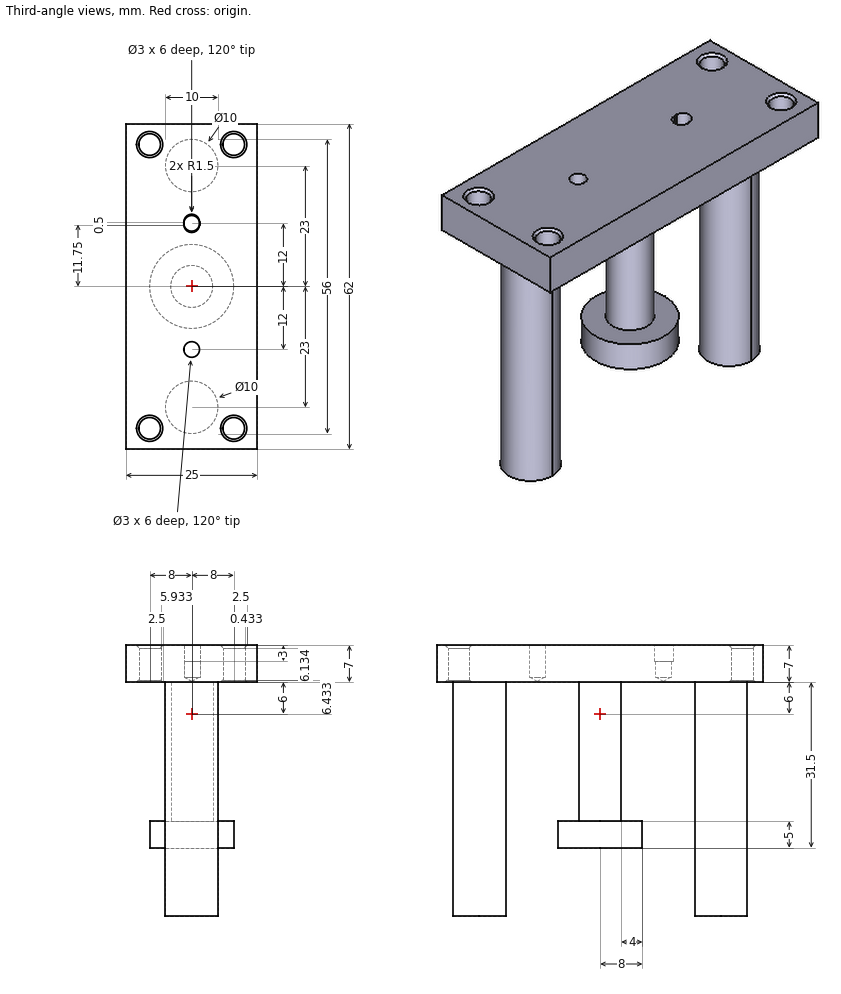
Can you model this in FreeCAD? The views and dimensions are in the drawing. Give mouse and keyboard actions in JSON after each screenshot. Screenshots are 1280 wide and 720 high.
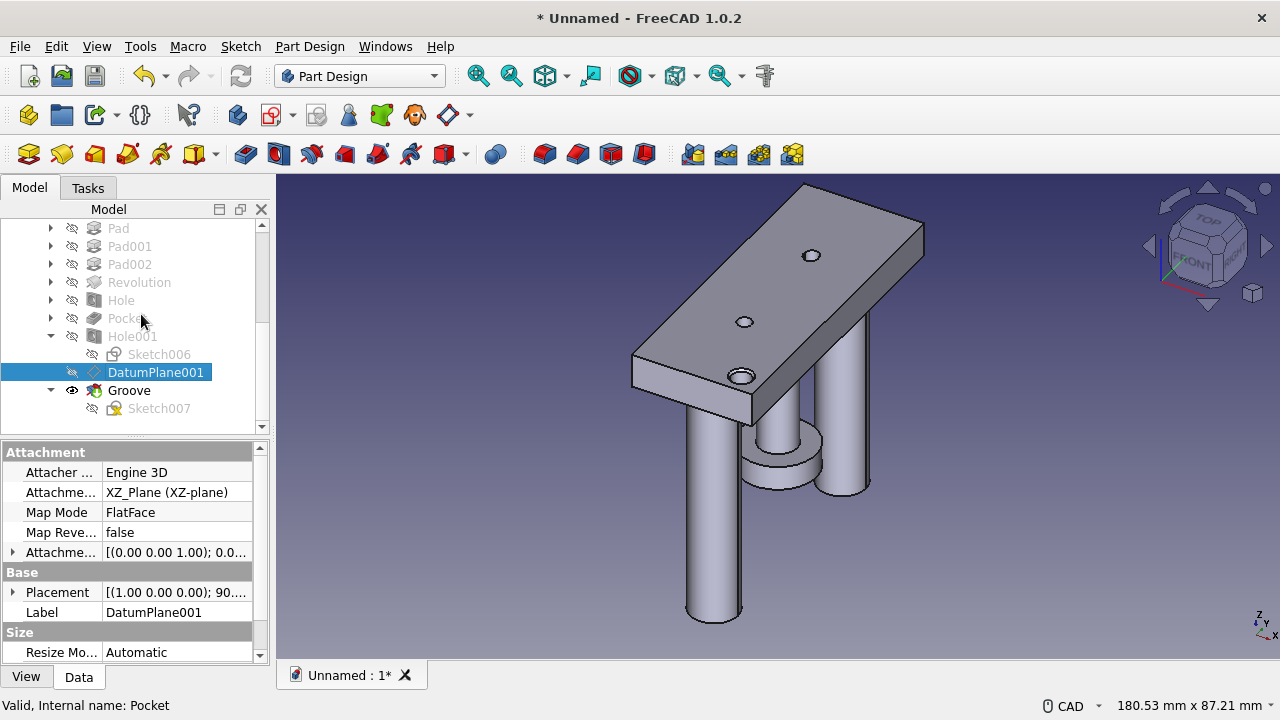
{"action": "scroll", "coordinate": [141, 314], "scroll_direction": "up", "scroll_amount": 15}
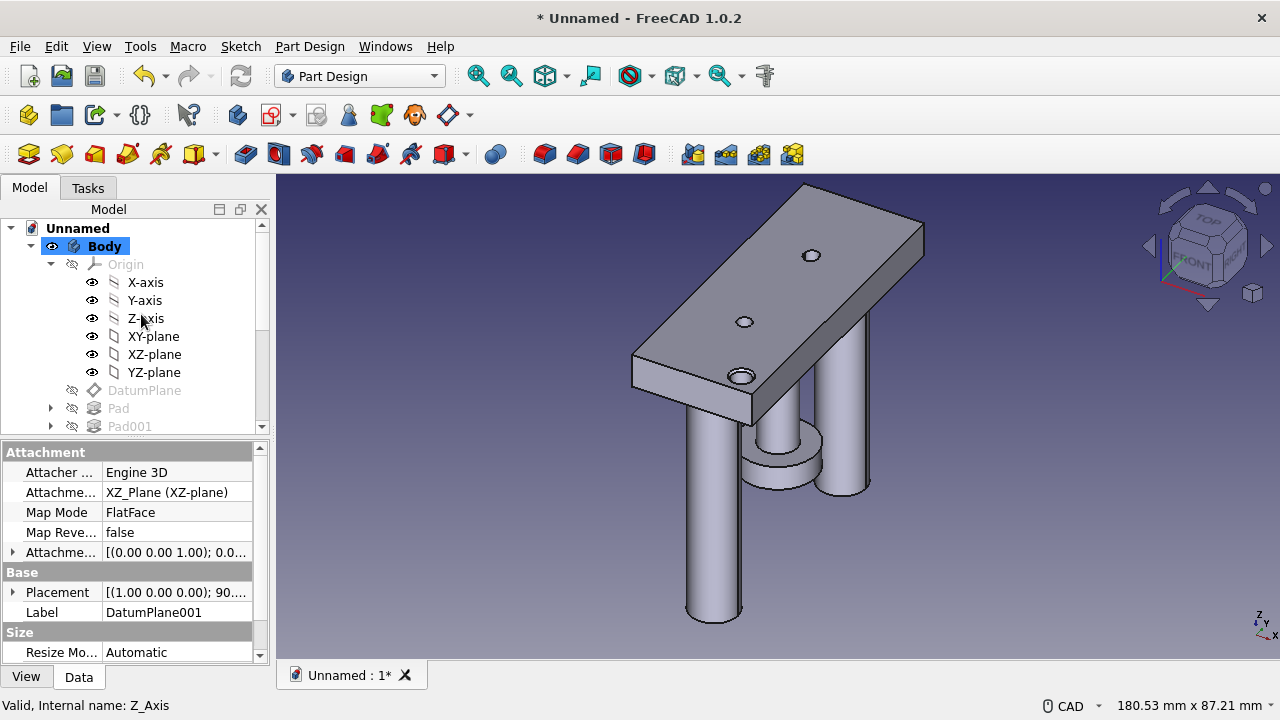
{"action": "left_click", "coordinate": [137, 354]}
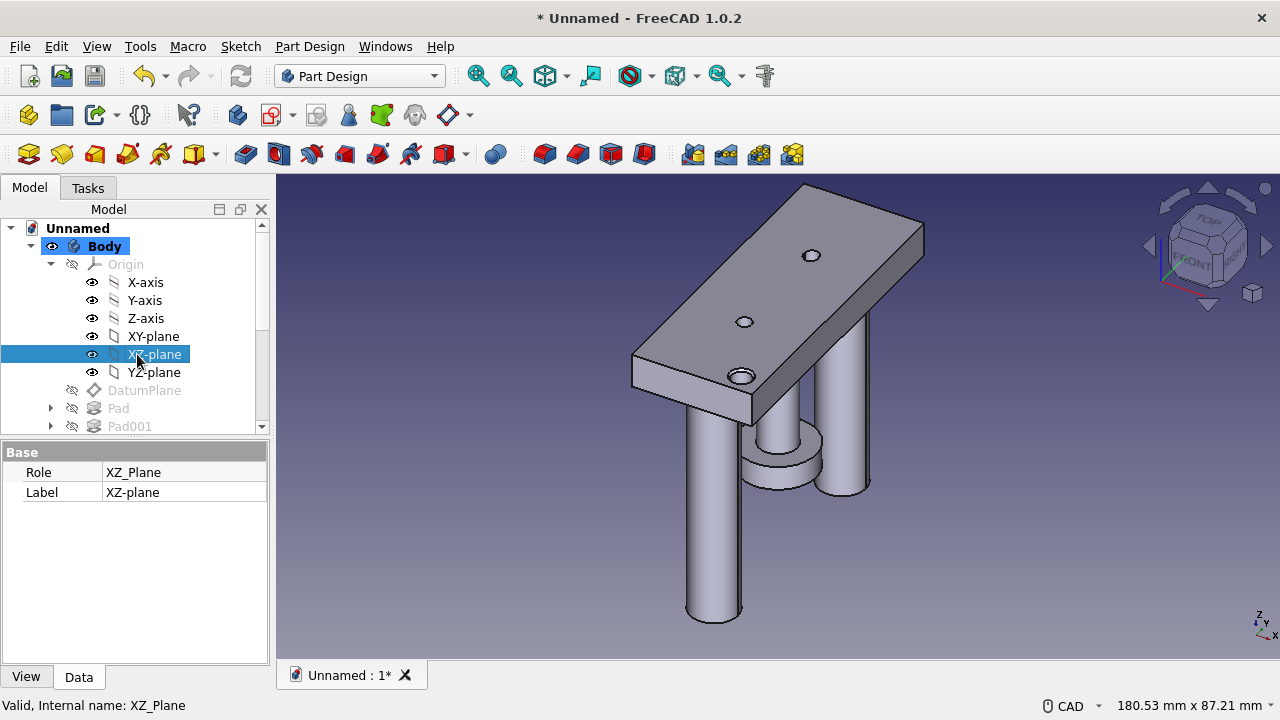
{"action": "left_click", "coordinate": [448, 116]}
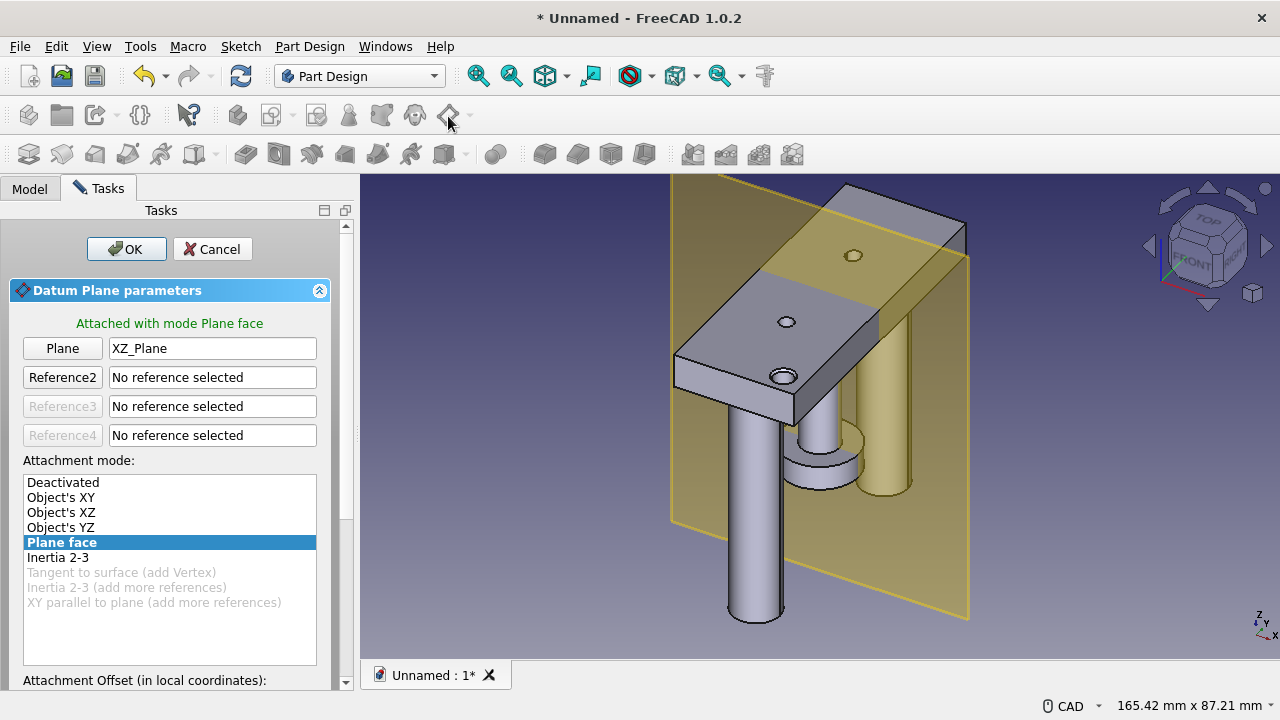
{"action": "scroll", "coordinate": [346, 455], "scroll_direction": "down", "scroll_amount": 3}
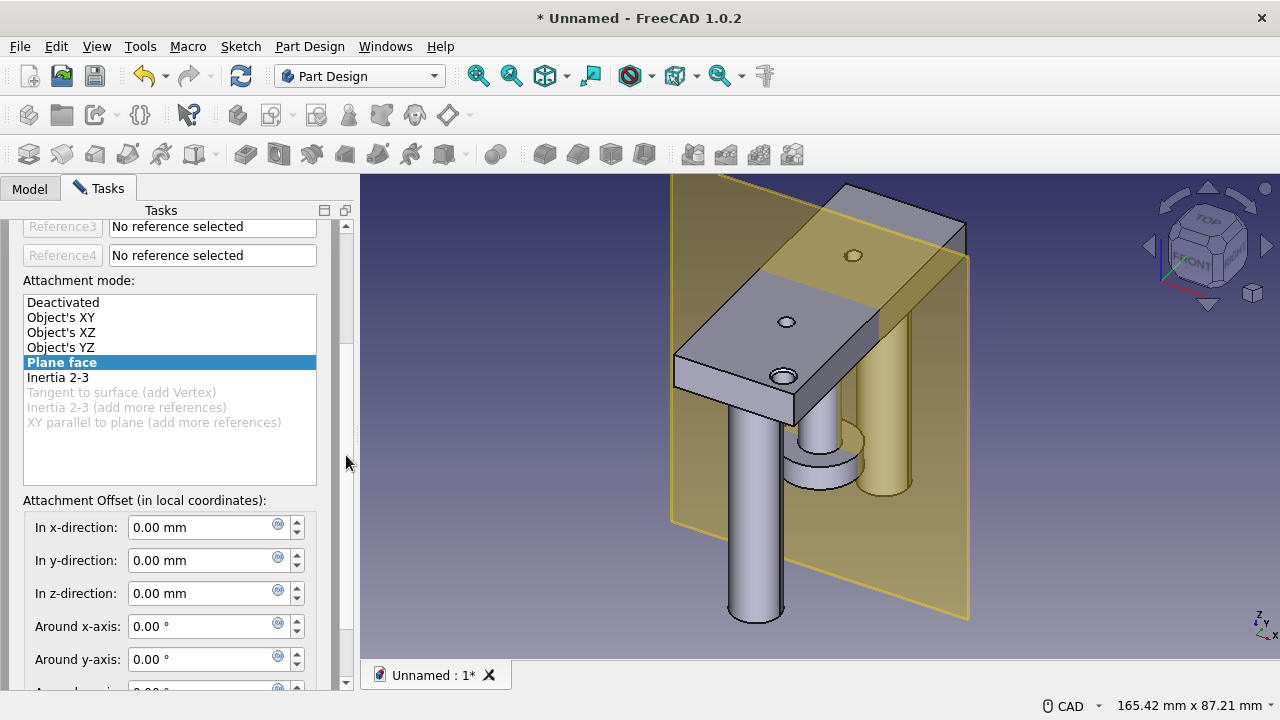
{"action": "triple_click", "coordinate": [210, 594]}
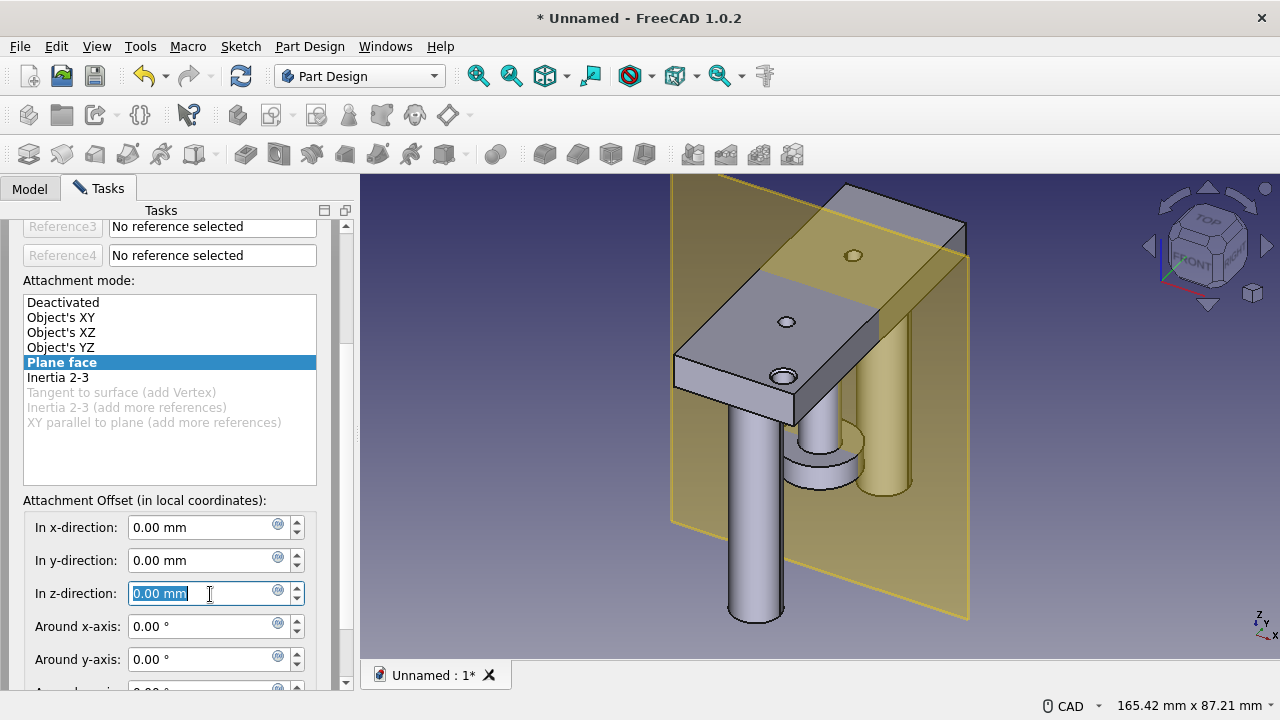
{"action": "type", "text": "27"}
{"action": "key", "text": "Tab"}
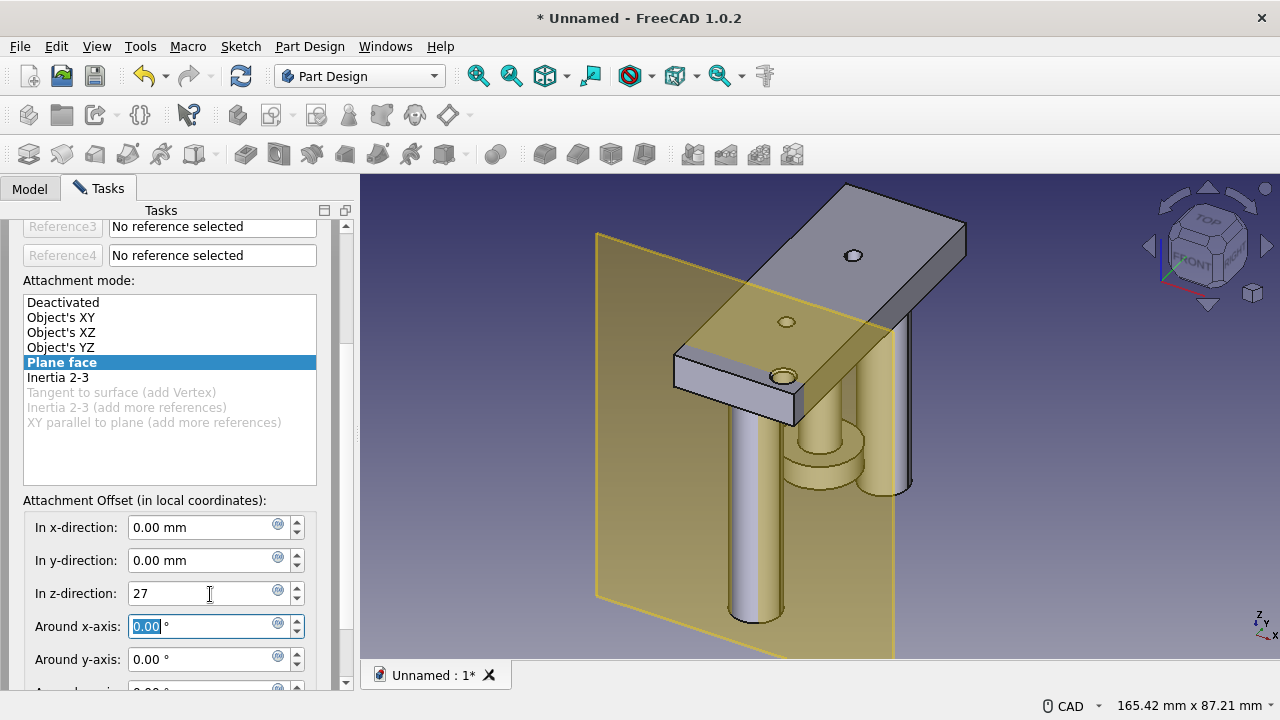
{"action": "scroll", "coordinate": [346, 455], "scroll_direction": "up", "scroll_amount": 4}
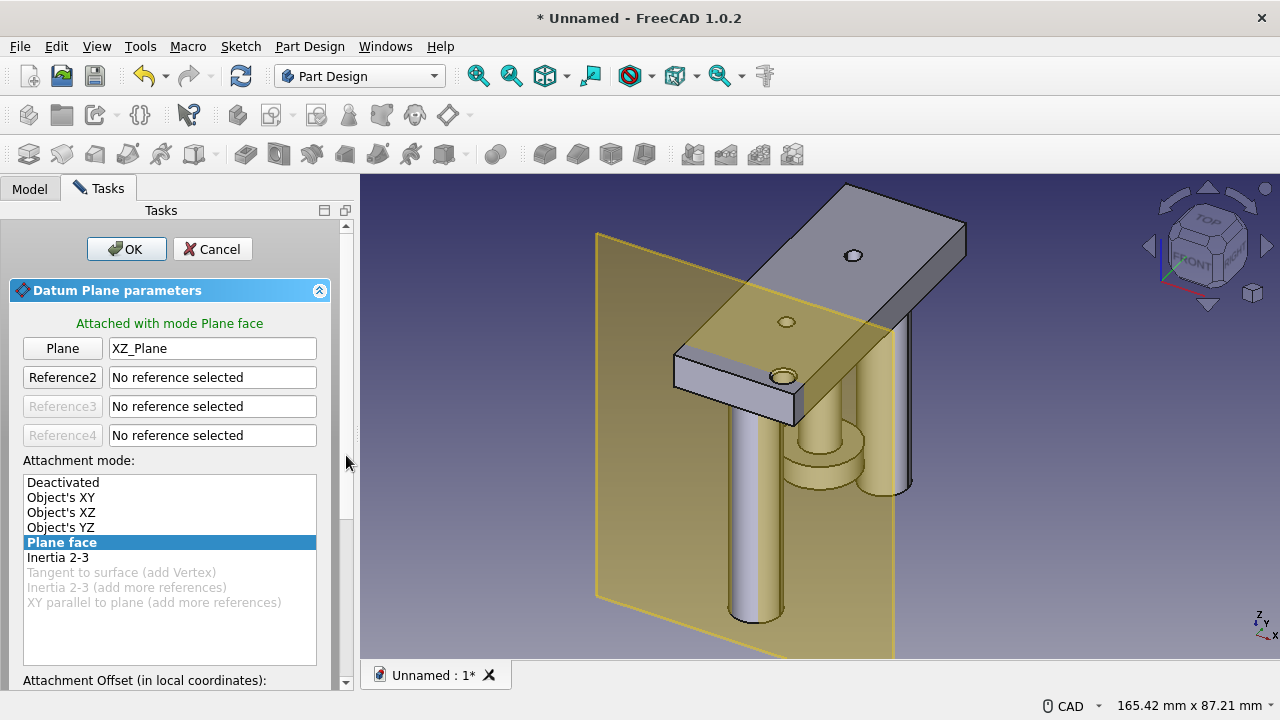
{"action": "left_click", "coordinate": [127, 249]}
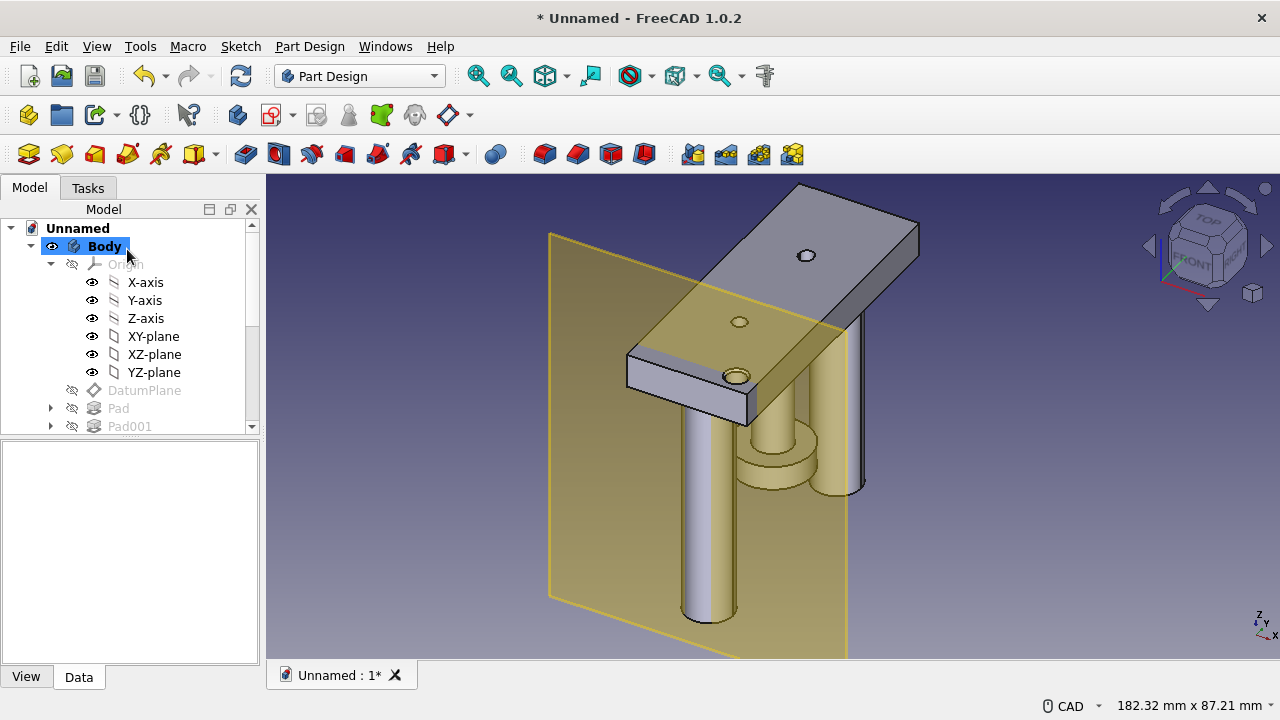
{"action": "scroll", "coordinate": [101, 332], "scroll_direction": "down", "scroll_amount": 3}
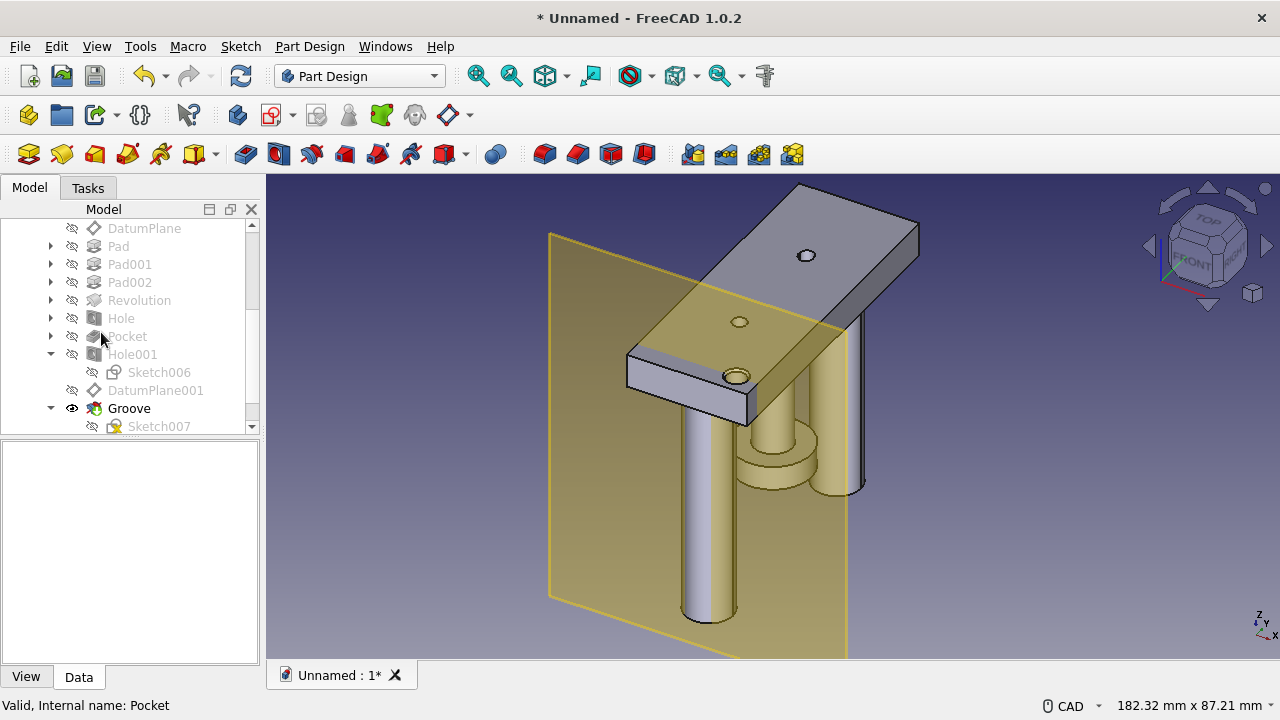
{"action": "scroll", "coordinate": [141, 332], "scroll_direction": "up", "scroll_amount": 15}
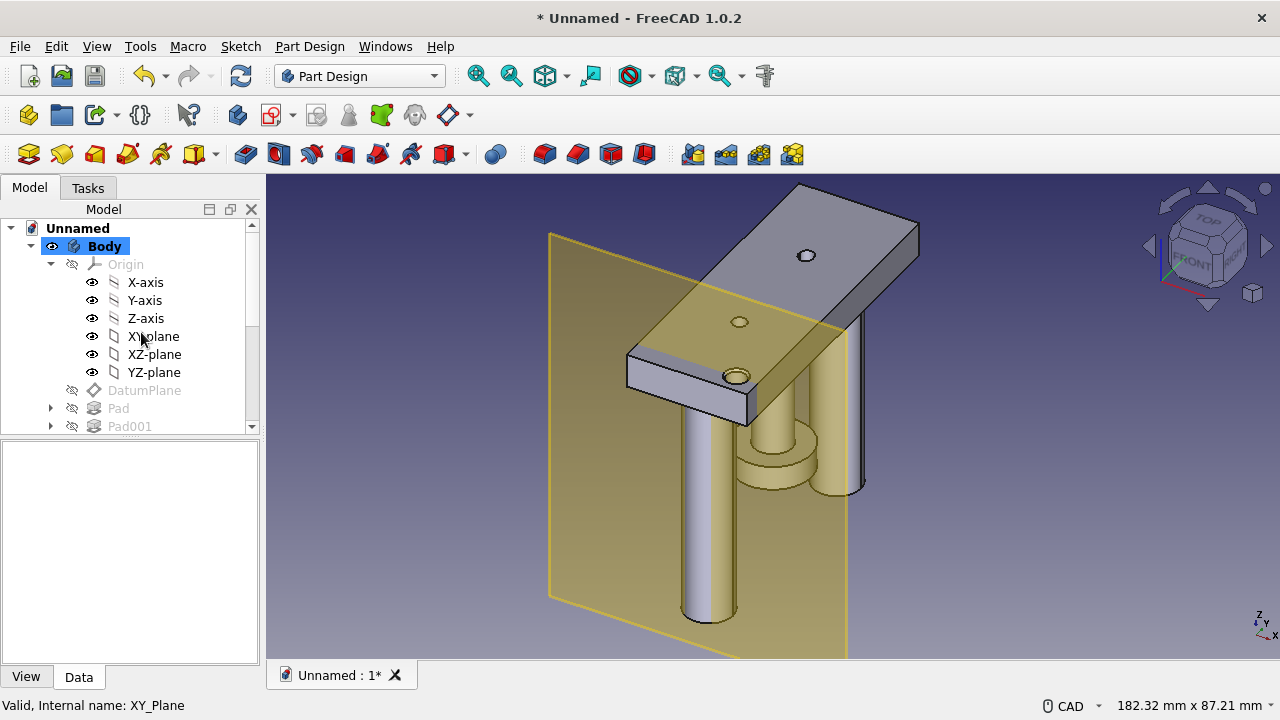
{"action": "scroll", "coordinate": [101, 332], "scroll_direction": "down", "scroll_amount": 6}